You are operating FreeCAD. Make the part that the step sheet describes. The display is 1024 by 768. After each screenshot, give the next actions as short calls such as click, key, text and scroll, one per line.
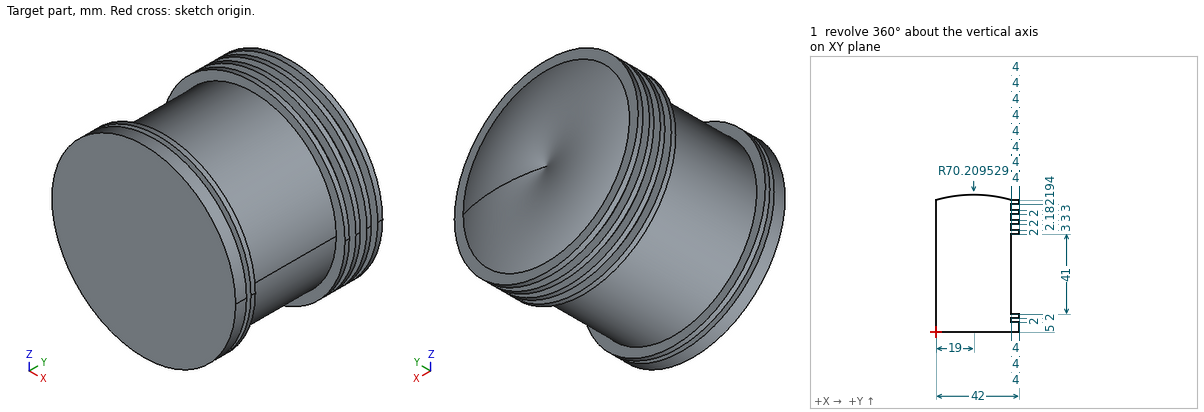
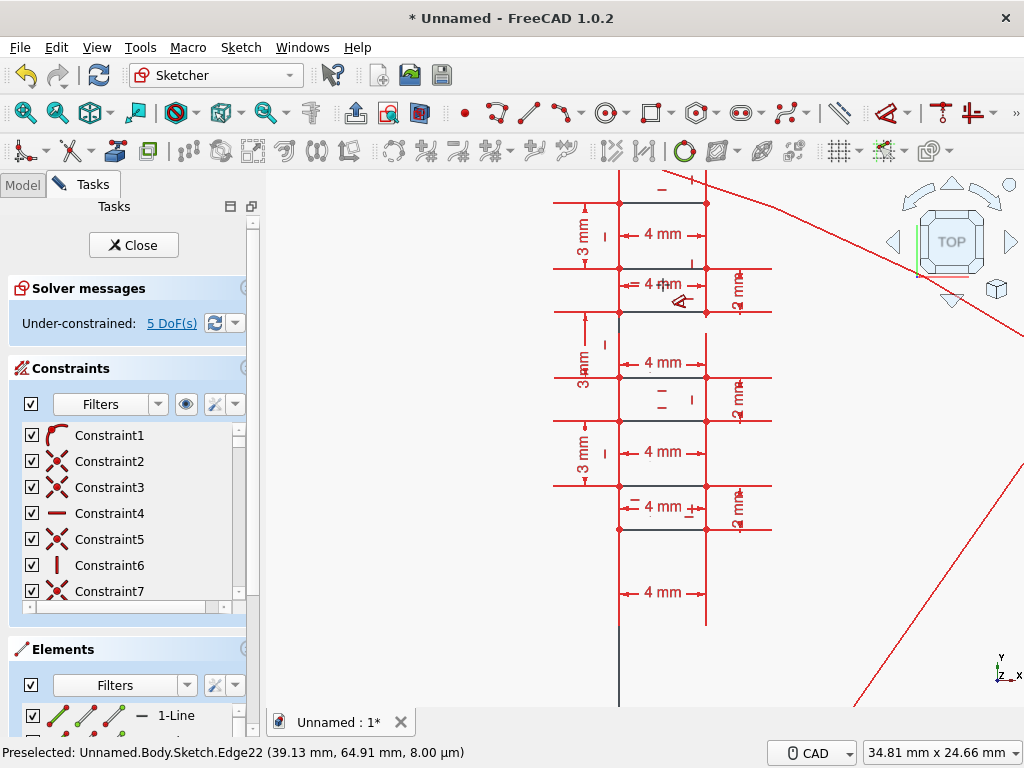
scroll(683, 302, down, 7)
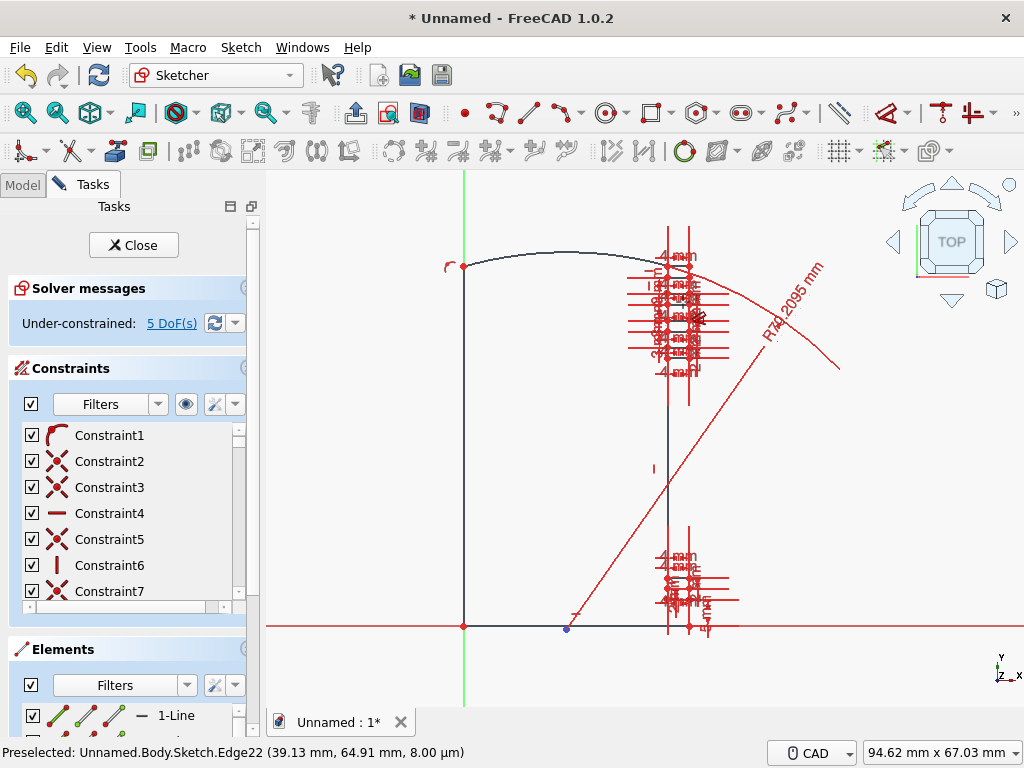
scroll(683, 266, up, 4)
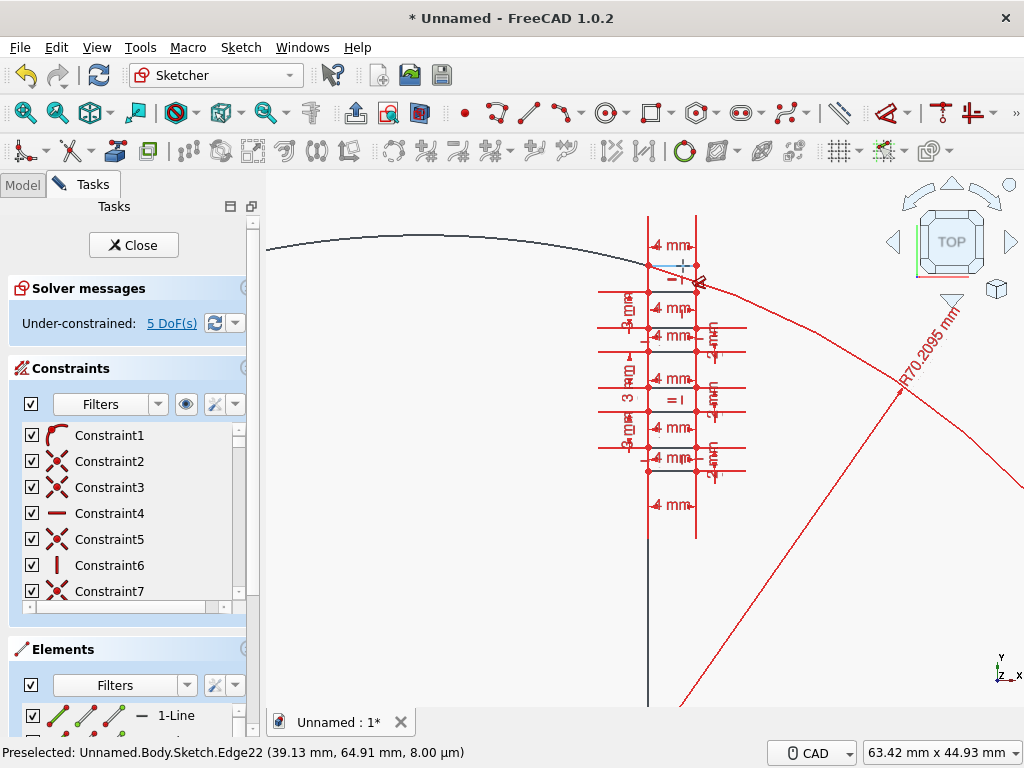
click(682, 266)
click(672, 208)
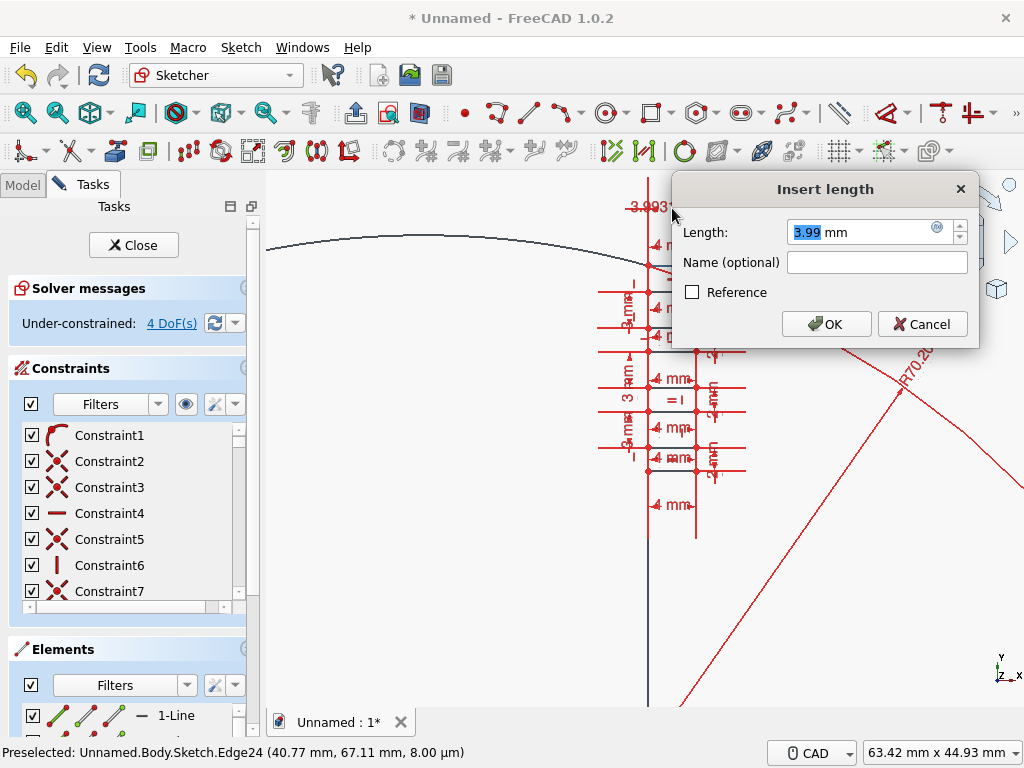
text(4)
key(Return)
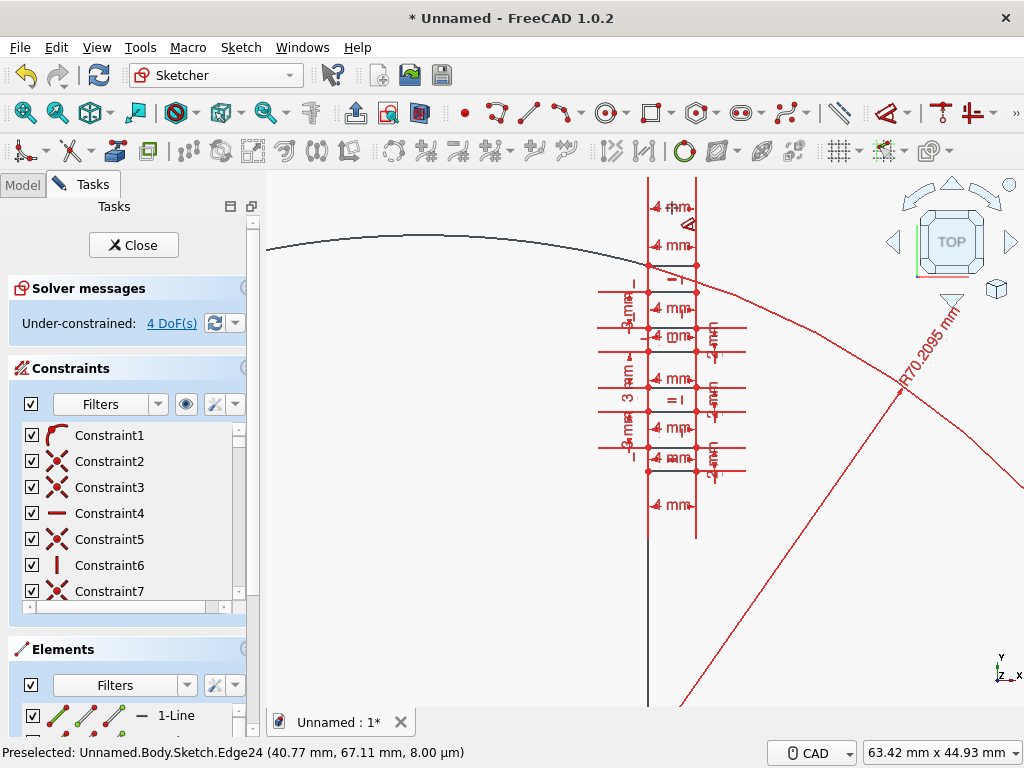
click(648, 618)
click(682, 575)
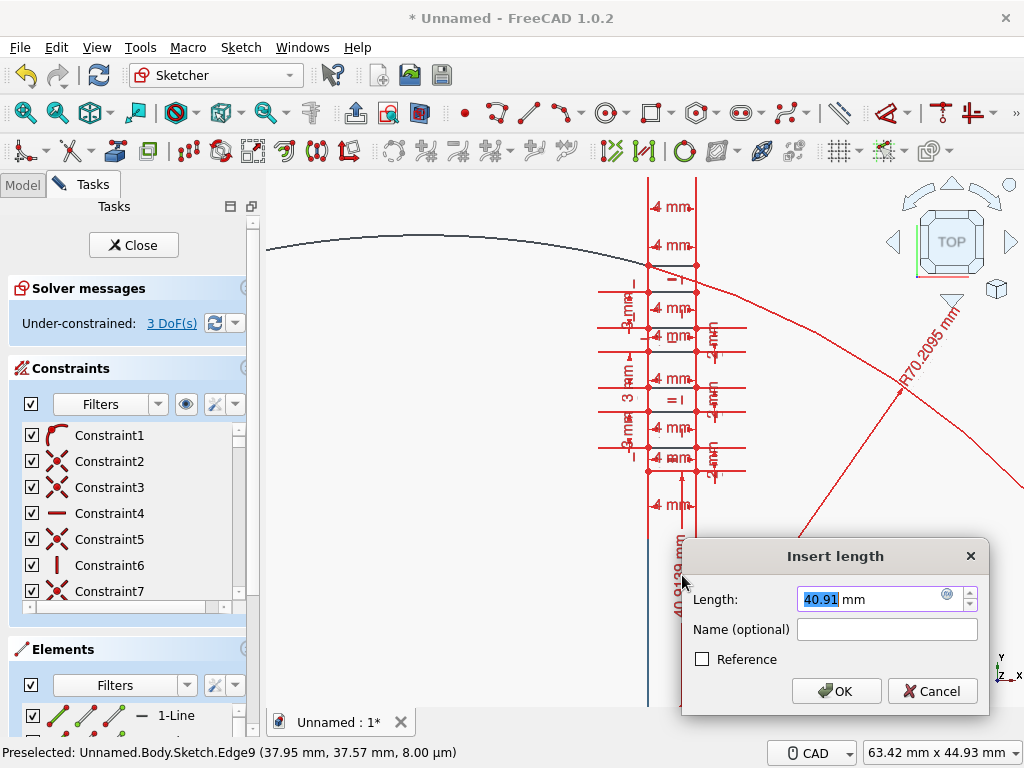
text(41)
key(Return)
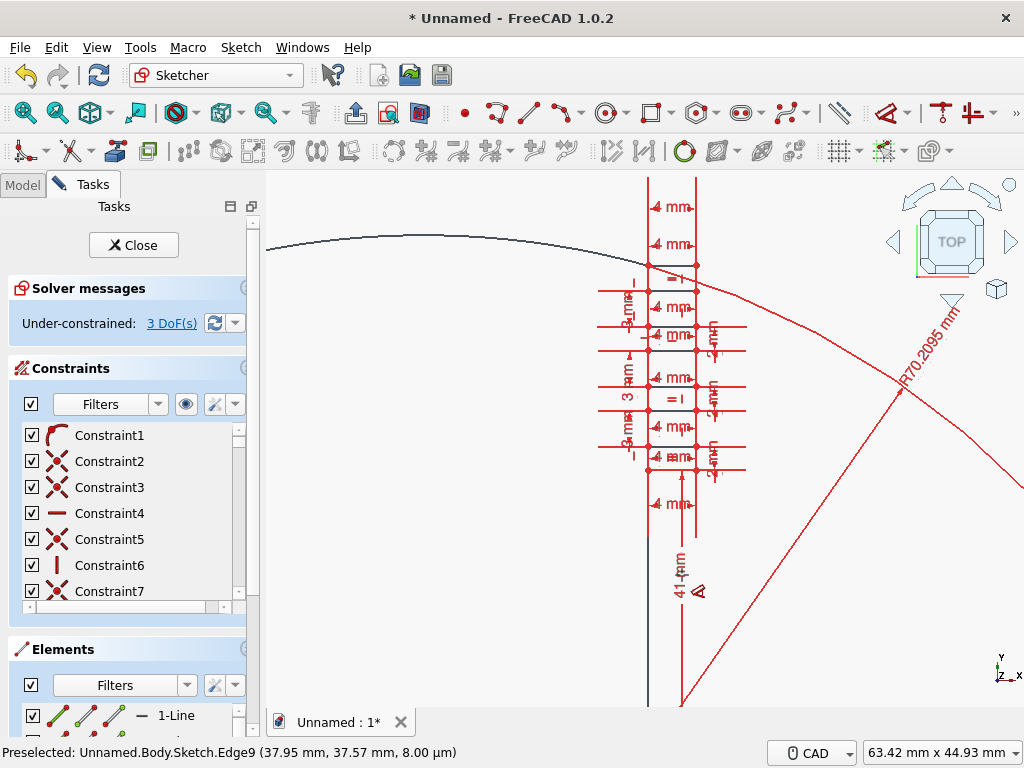
scroll(683, 265, down, 4)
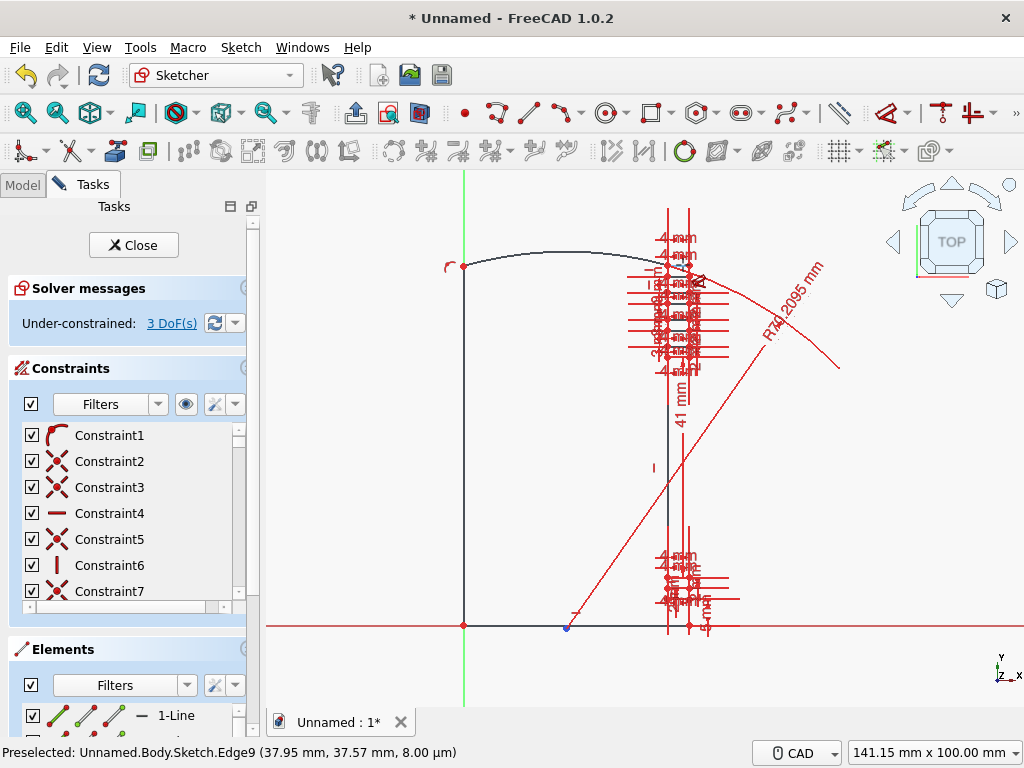
click(689, 626)
click(577, 660)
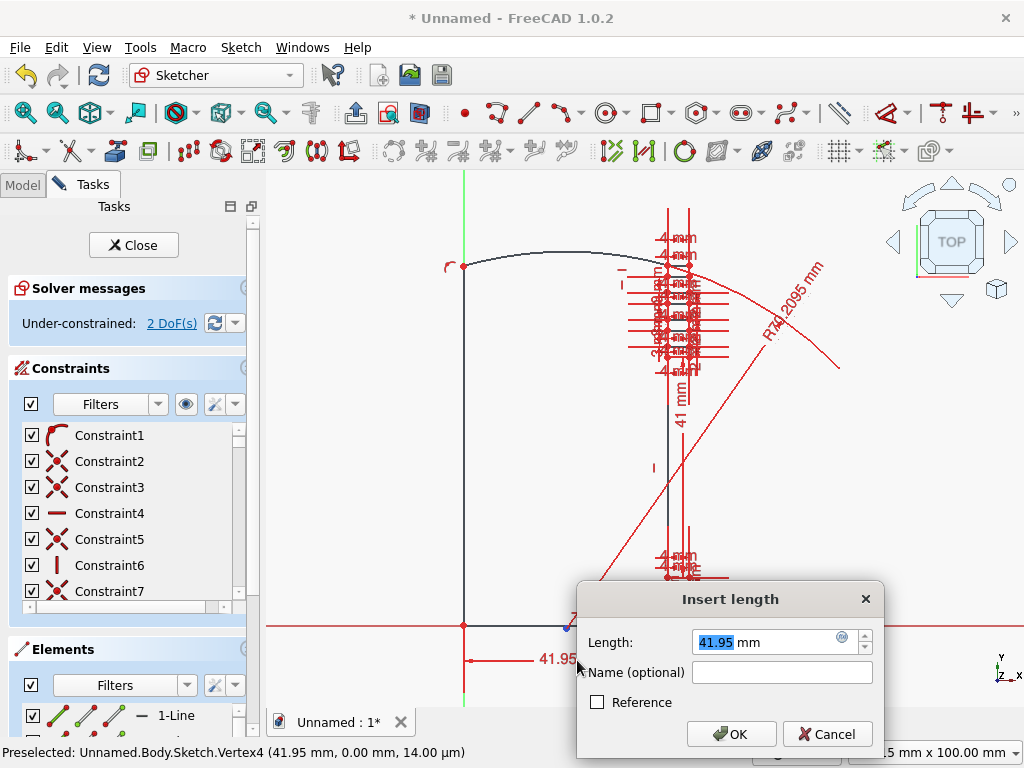
text(42)
key(Return)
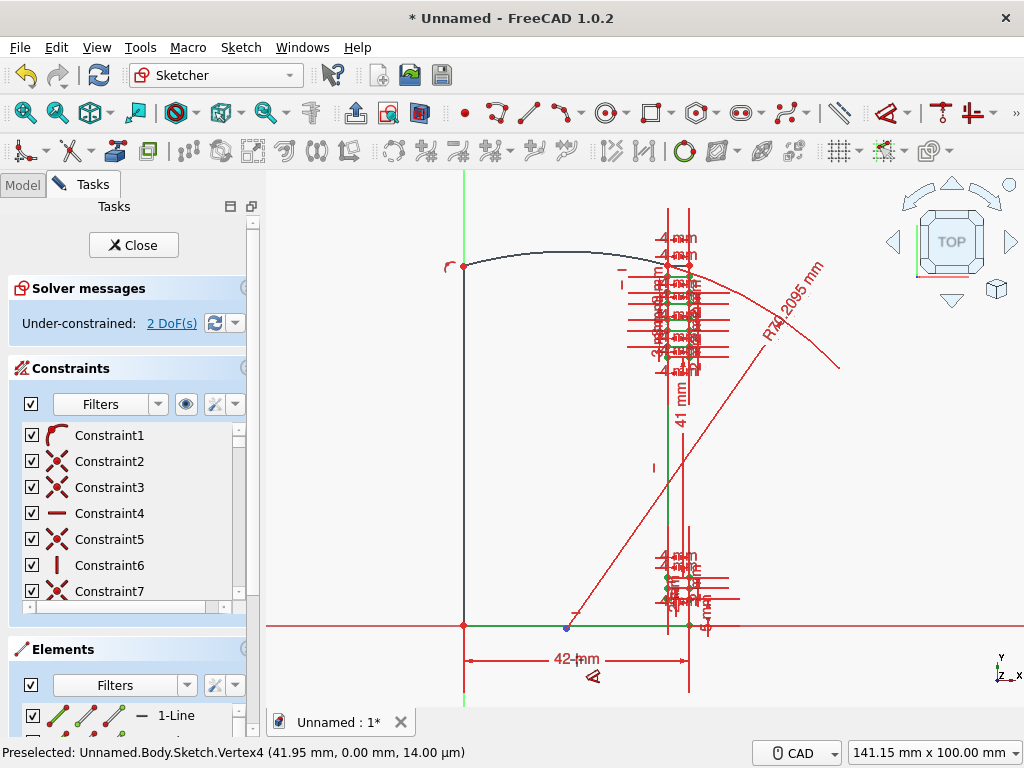
click(567, 629)
click(492, 663)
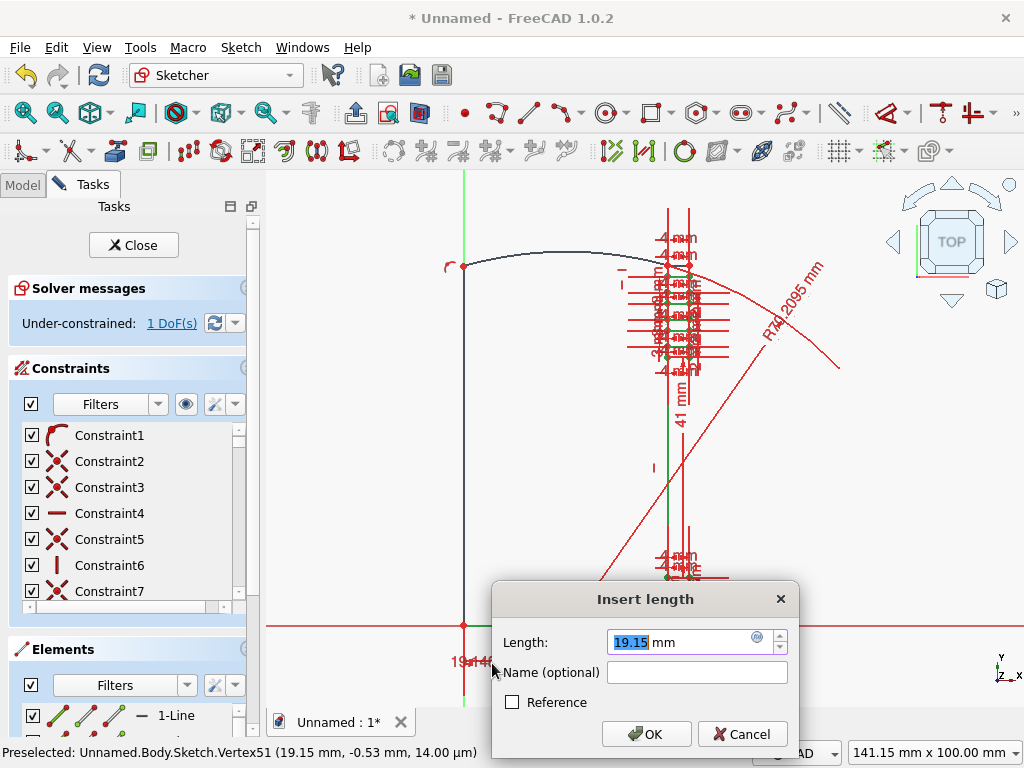
text(19)
key(Return)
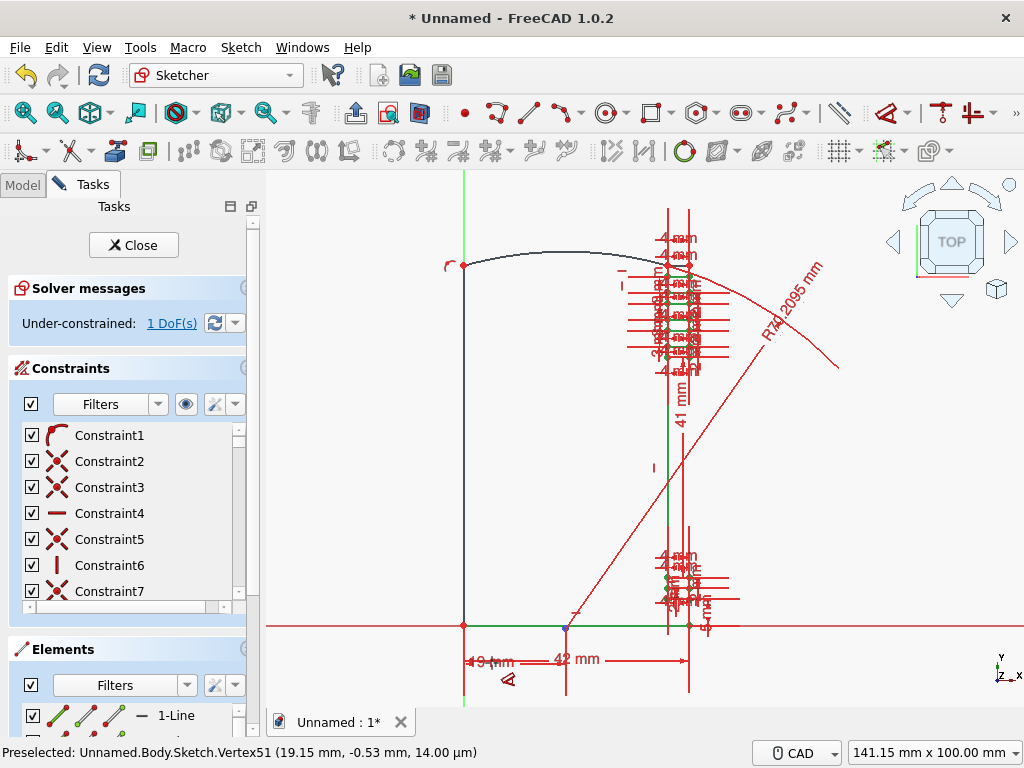
scroll(689, 271, up, 7)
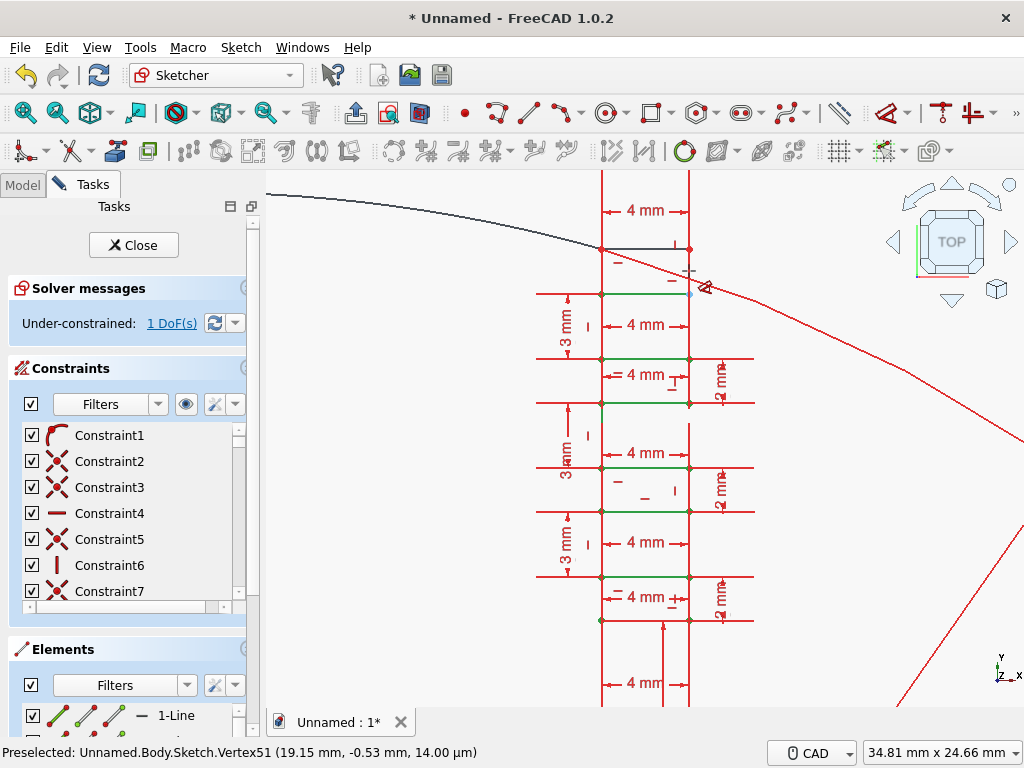
click(689, 272)
click(723, 272)